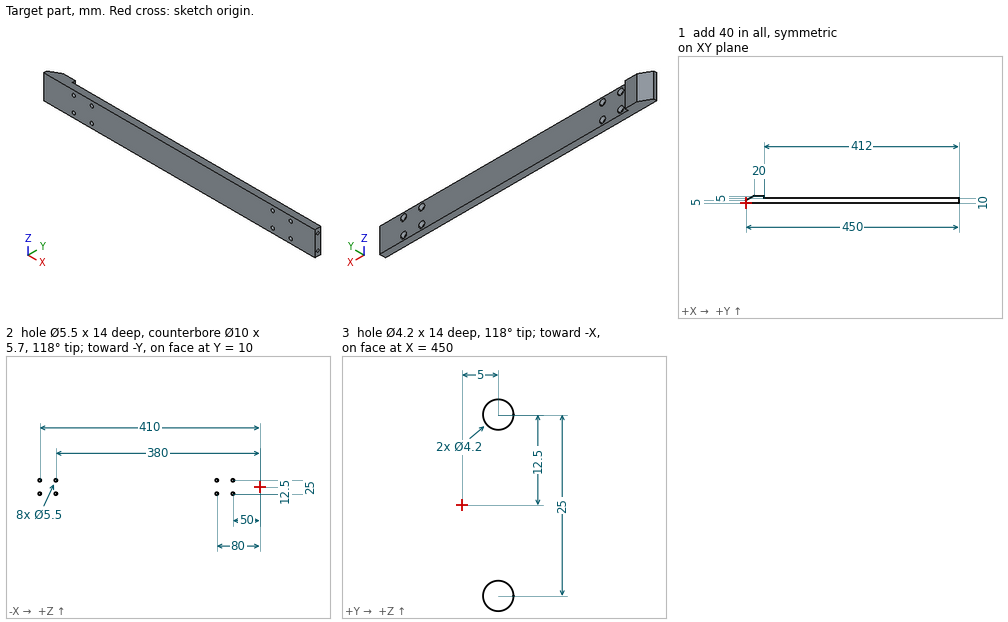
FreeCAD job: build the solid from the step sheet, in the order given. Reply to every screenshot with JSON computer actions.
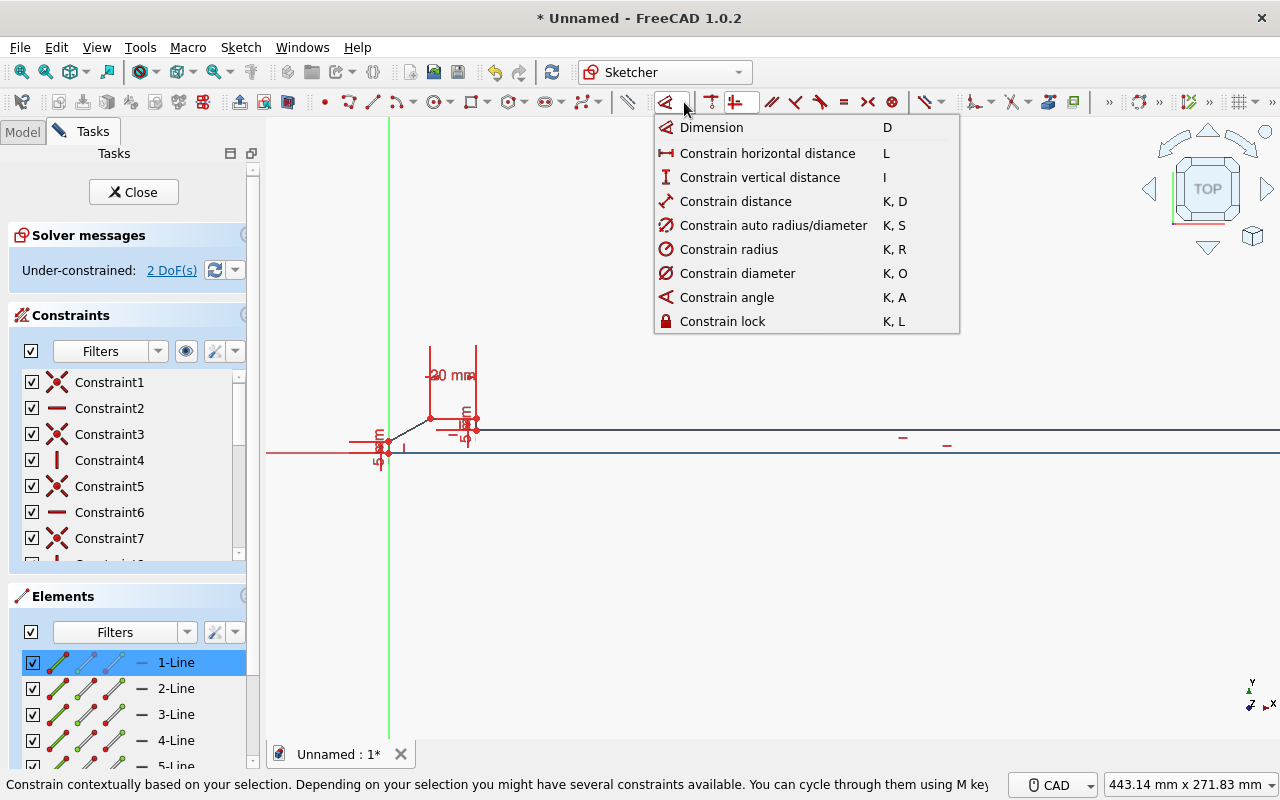
{"action": "left_click", "coordinate": [807, 153]}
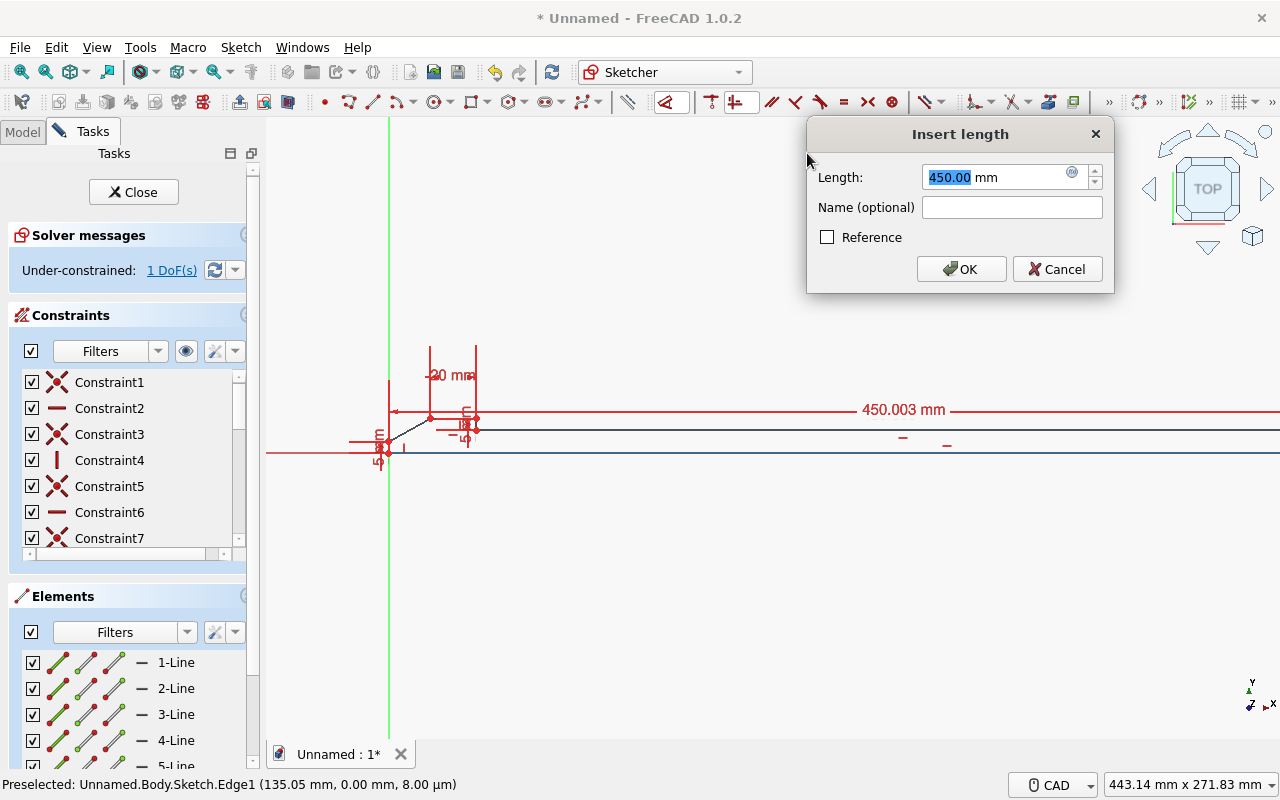
{"action": "type", "text": "450"}
{"action": "key", "text": "Return"}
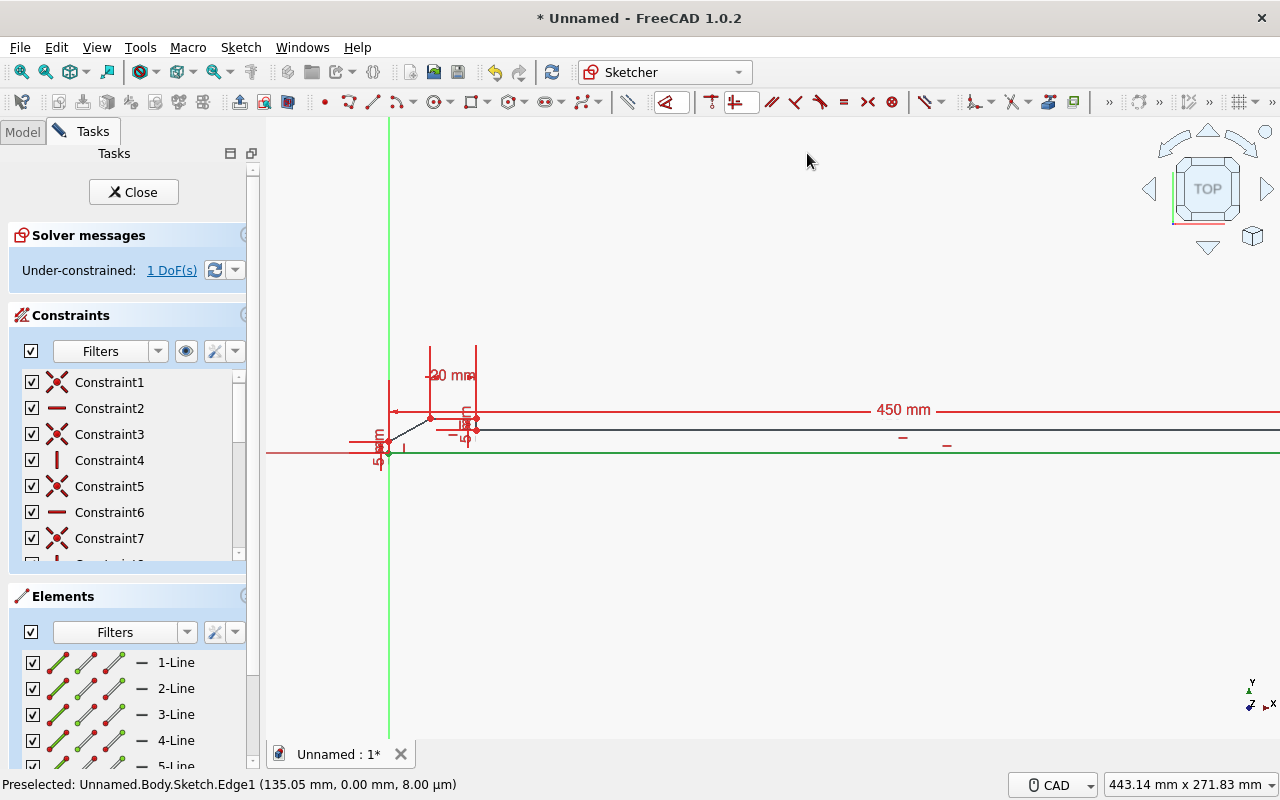
{"action": "left_click", "coordinate": [759, 430]}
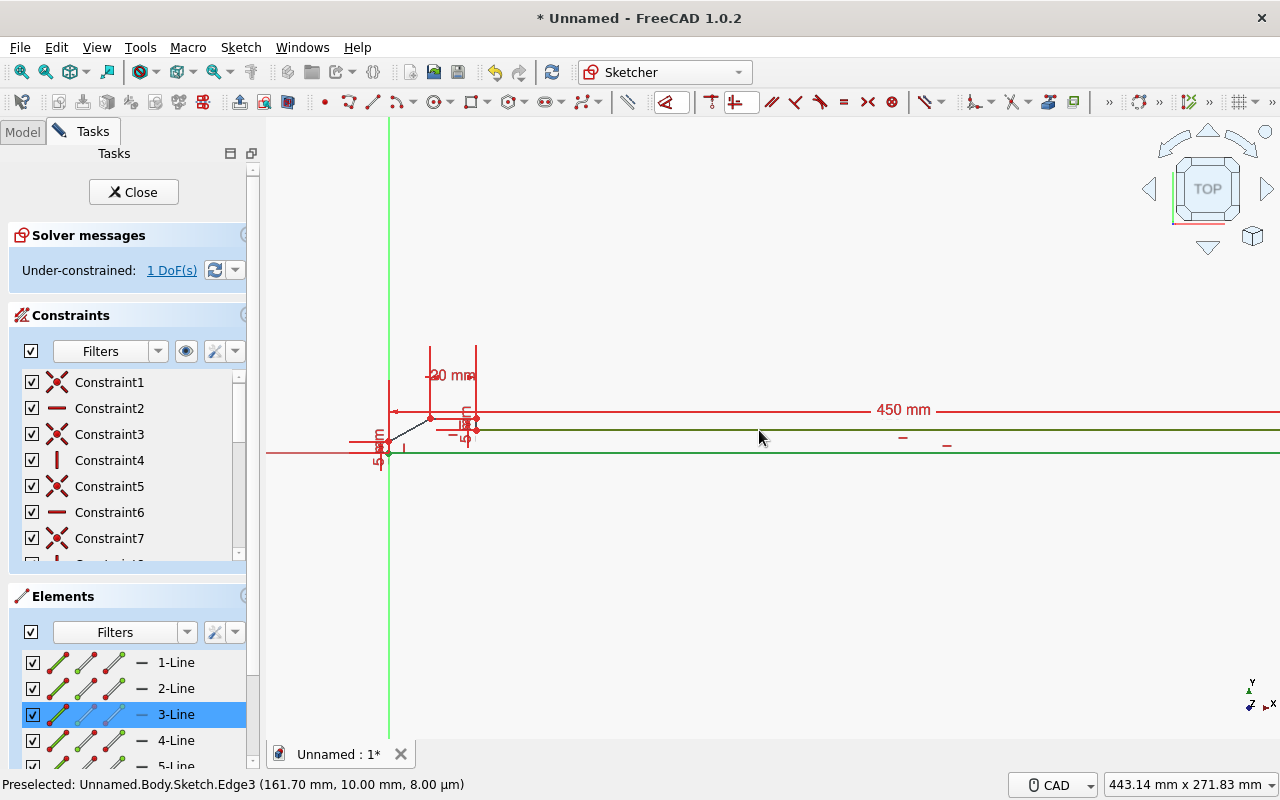
{"action": "key", "text": "l"}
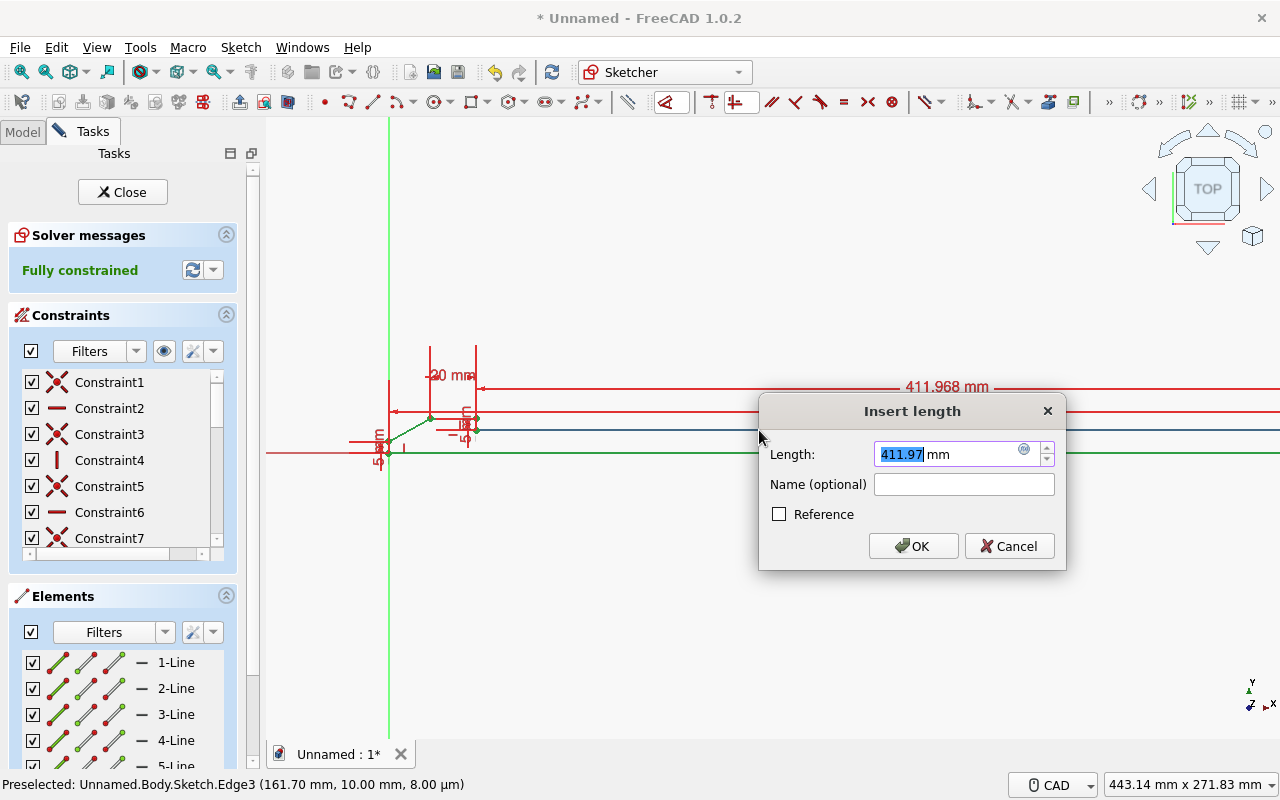
{"action": "type", "text": "412"}
{"action": "key", "text": "Return"}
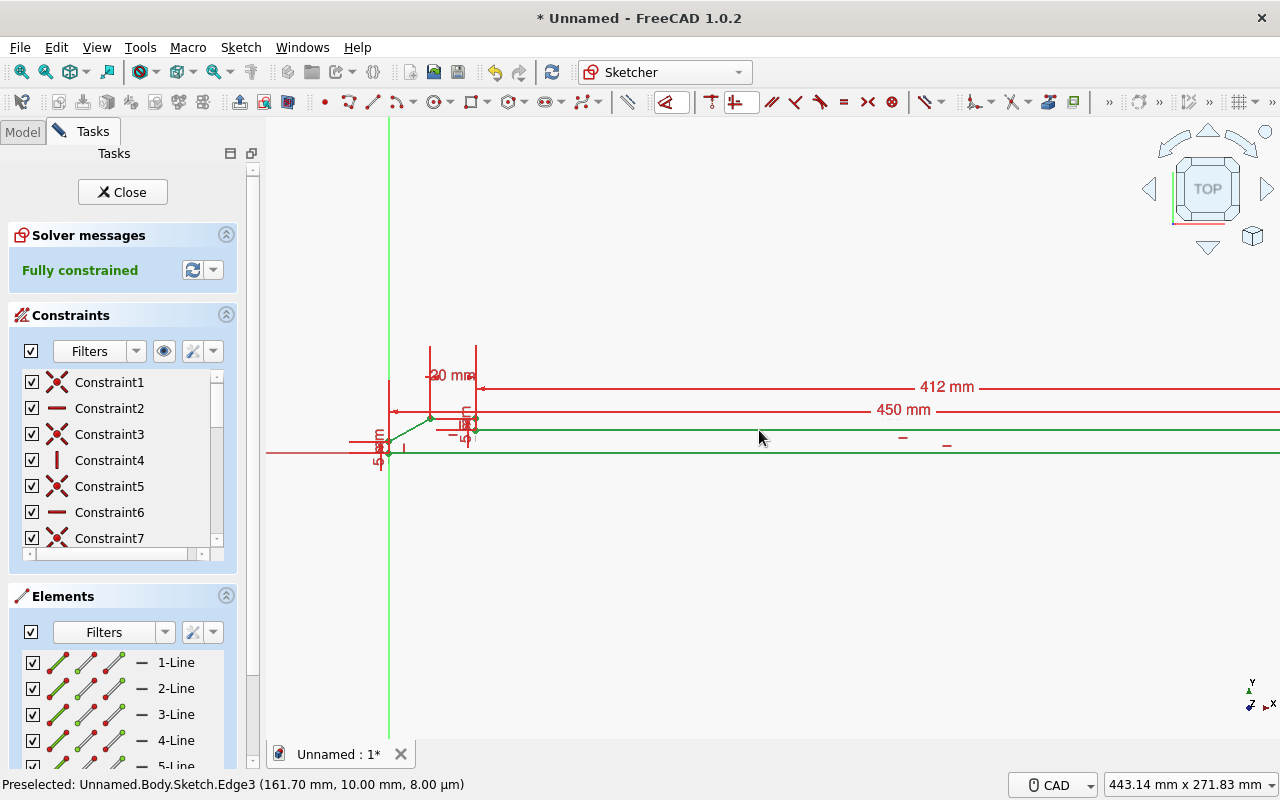
{"action": "left_click", "coordinate": [123, 192]}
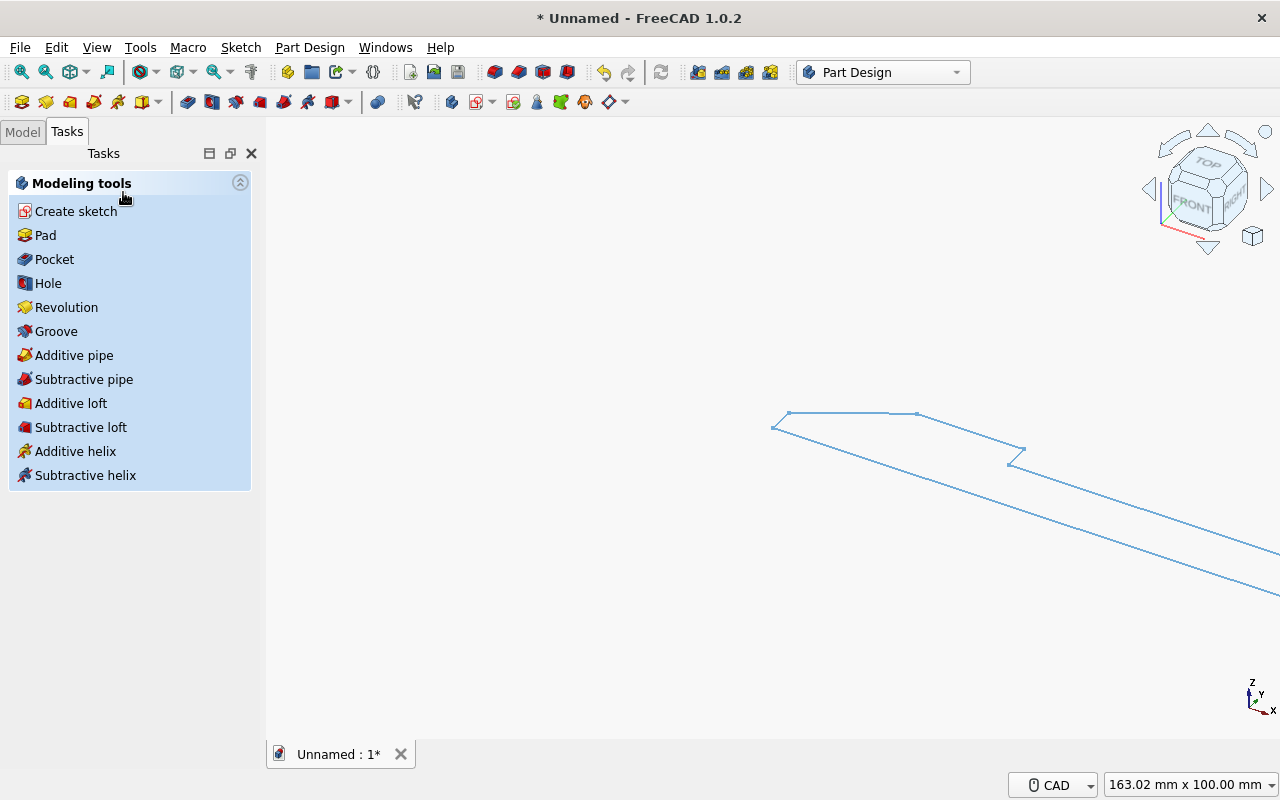
{"action": "left_click", "coordinate": [22, 102]}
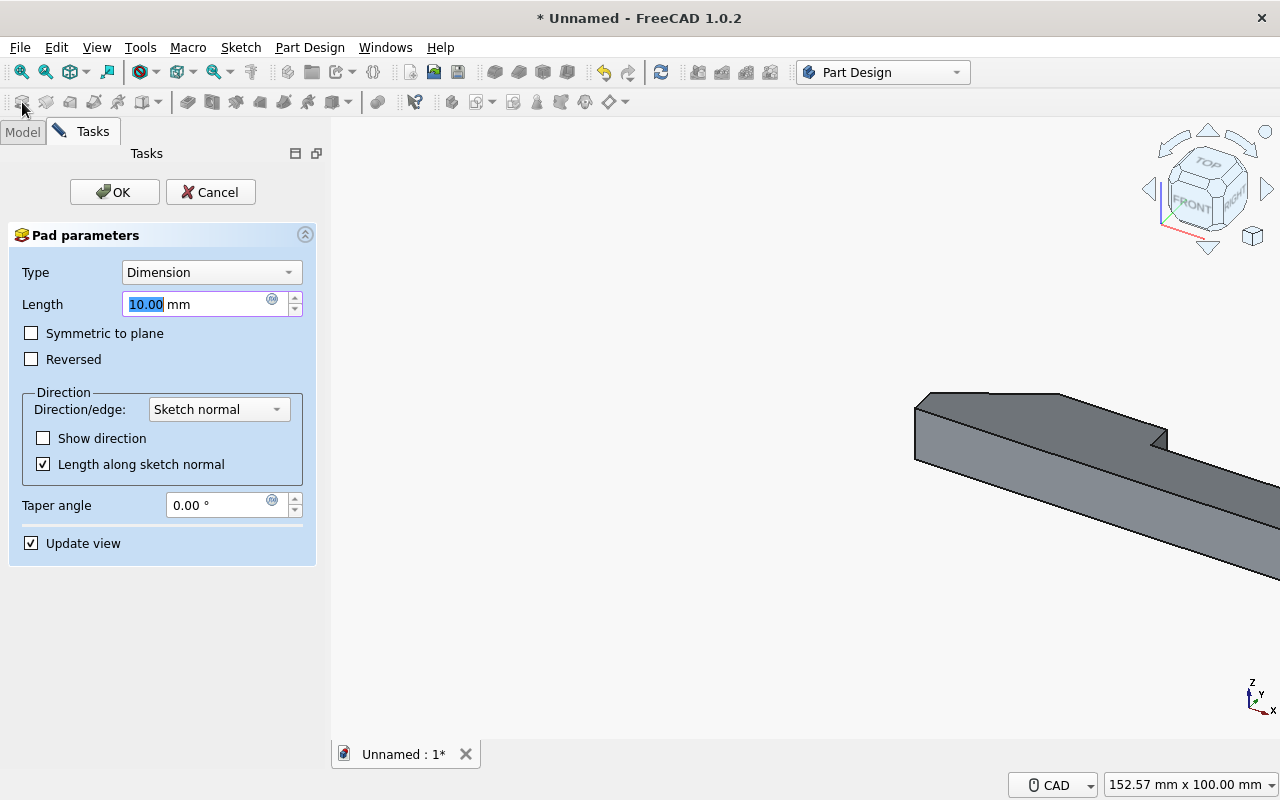
{"action": "type", "text": "40"}
{"action": "key", "text": "Tab"}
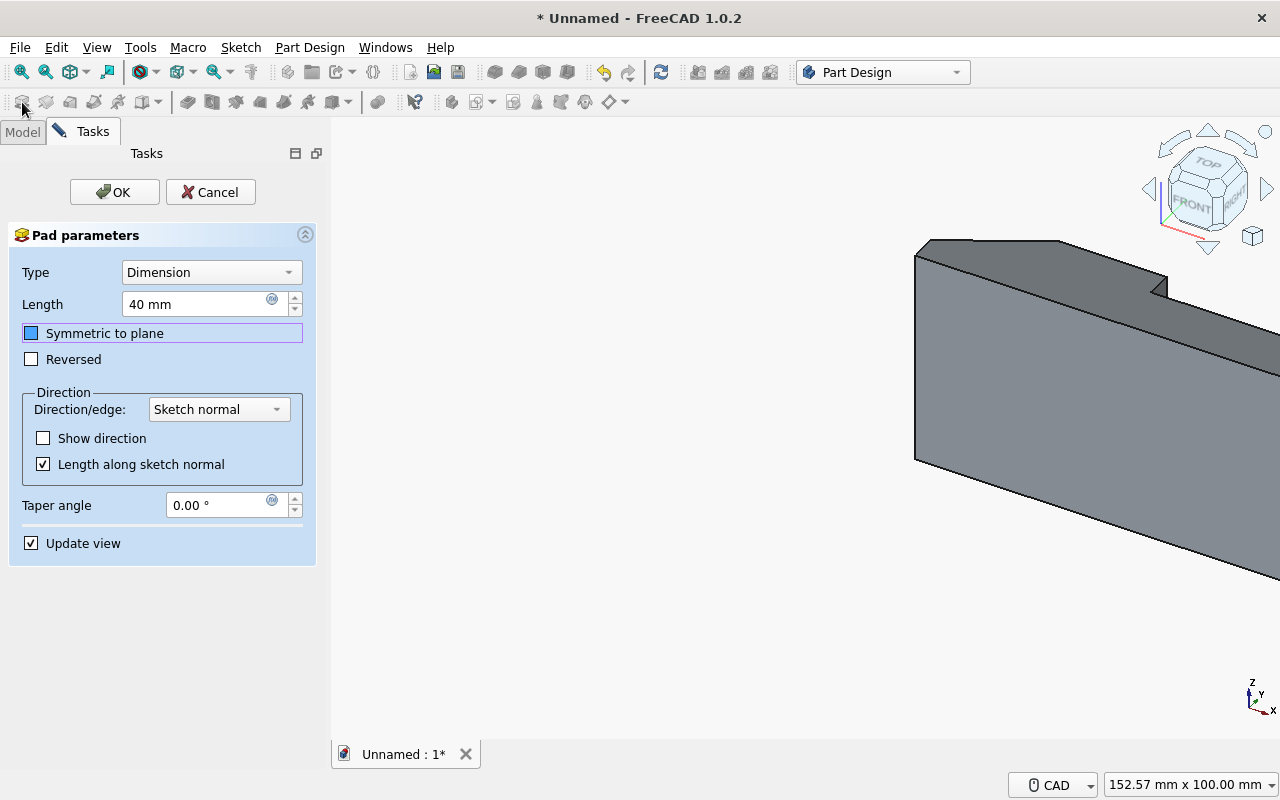
{"action": "left_click", "coordinate": [30, 333]}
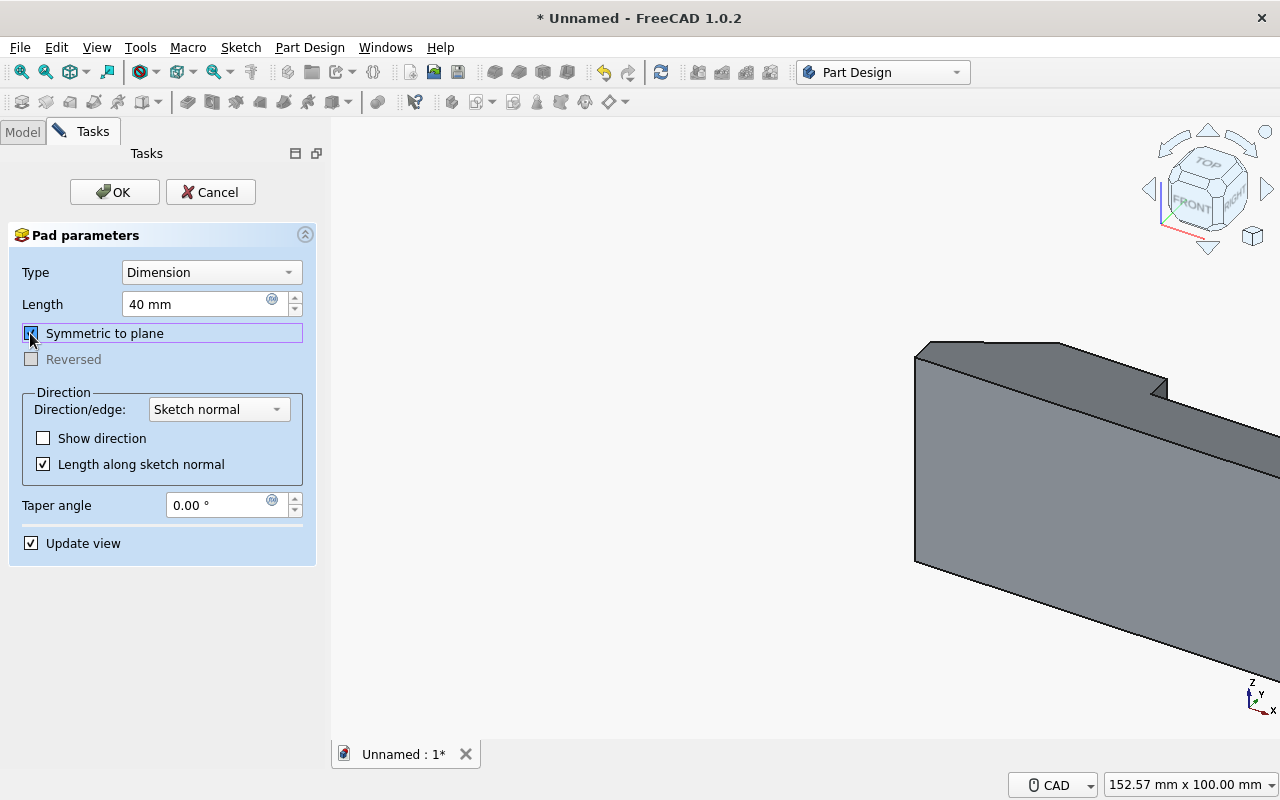
{"action": "left_click", "coordinate": [115, 192]}